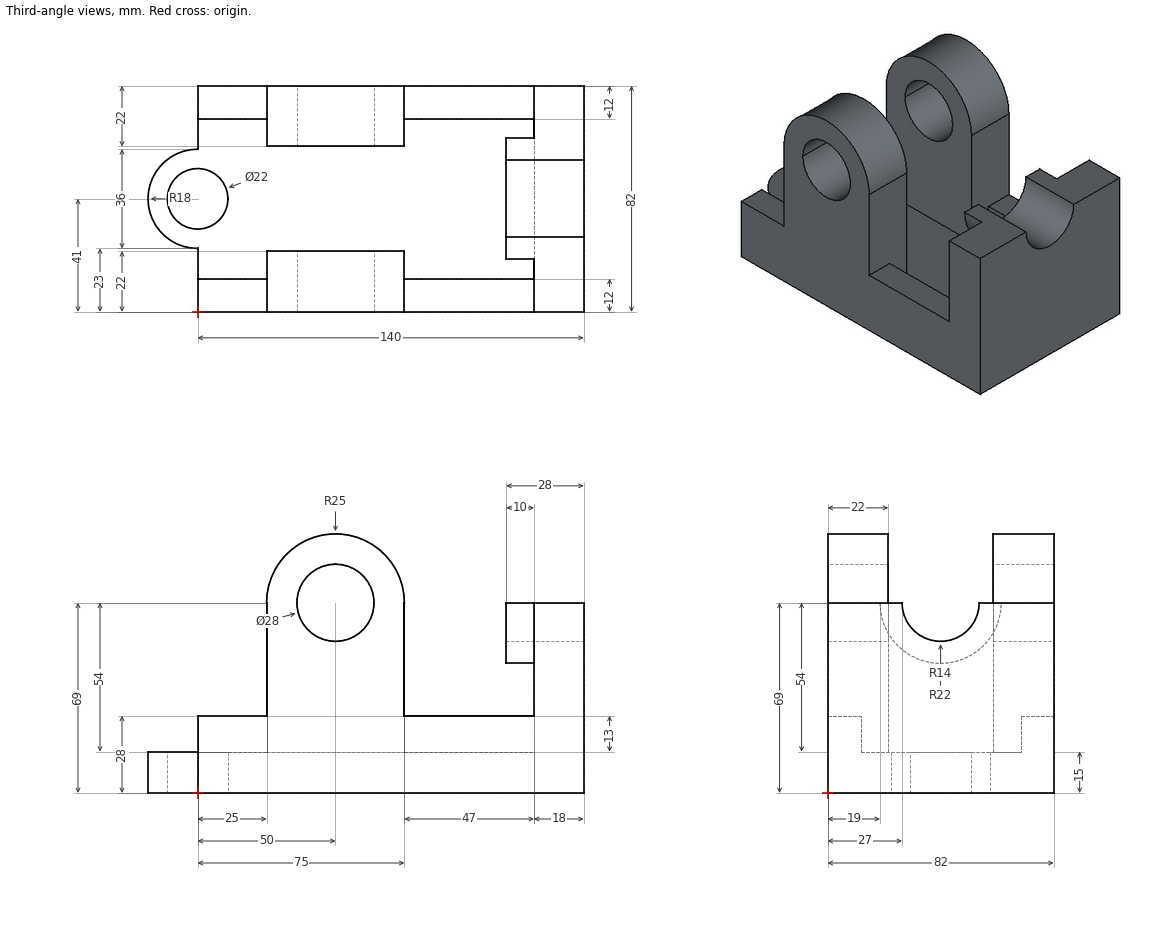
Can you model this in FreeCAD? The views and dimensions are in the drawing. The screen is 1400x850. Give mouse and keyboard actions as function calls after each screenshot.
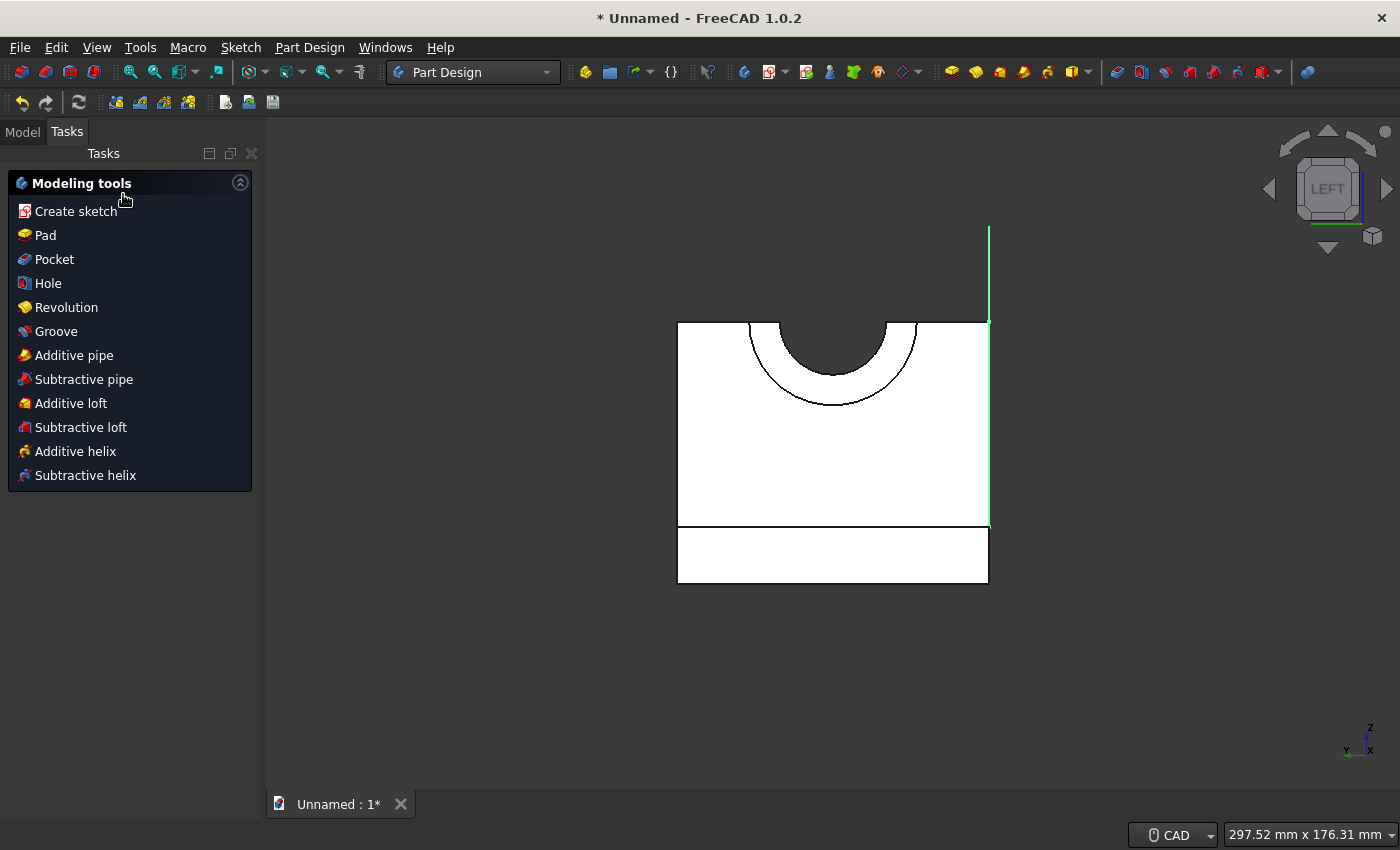
click(952, 72)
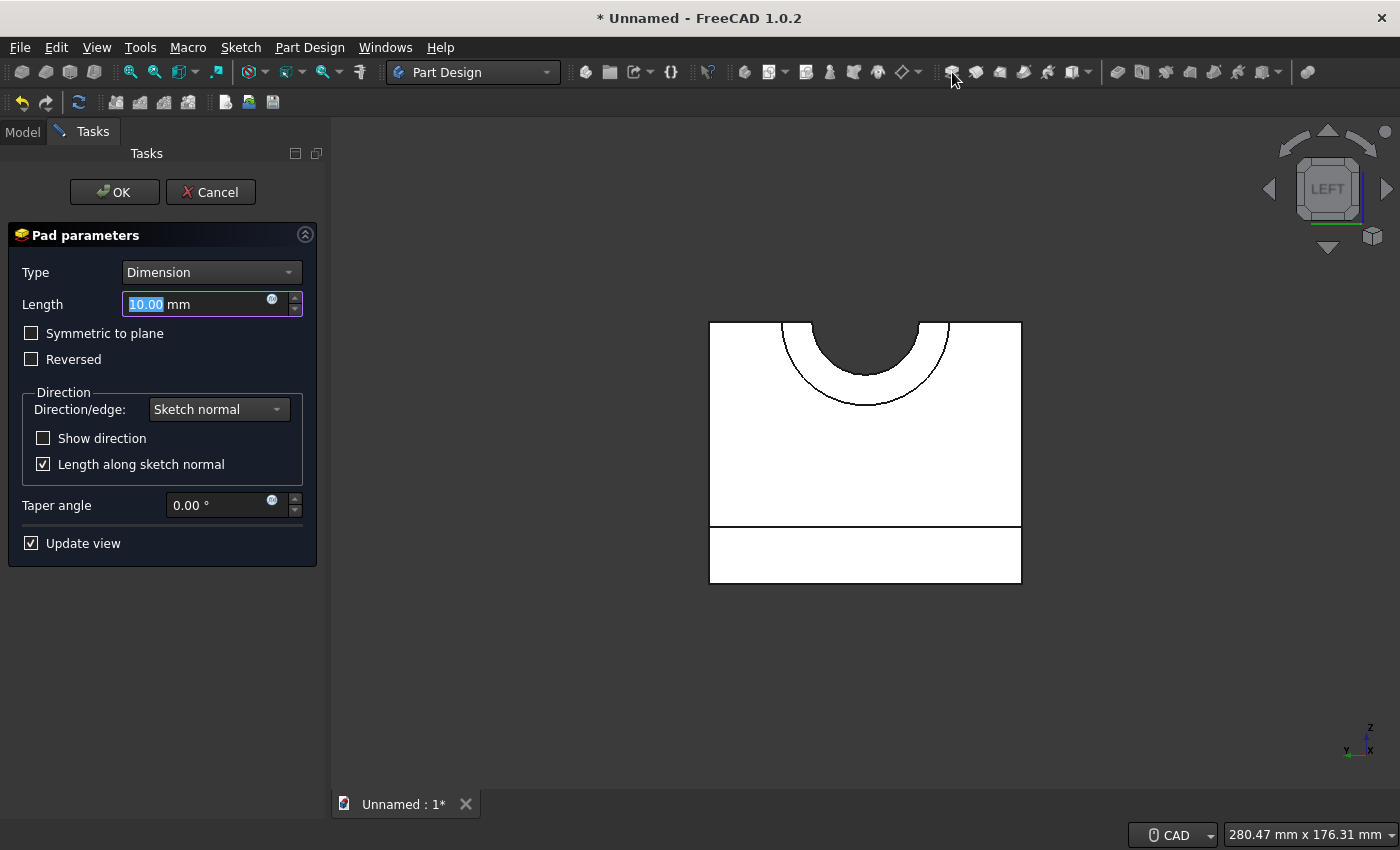
text(22)
key(Tab)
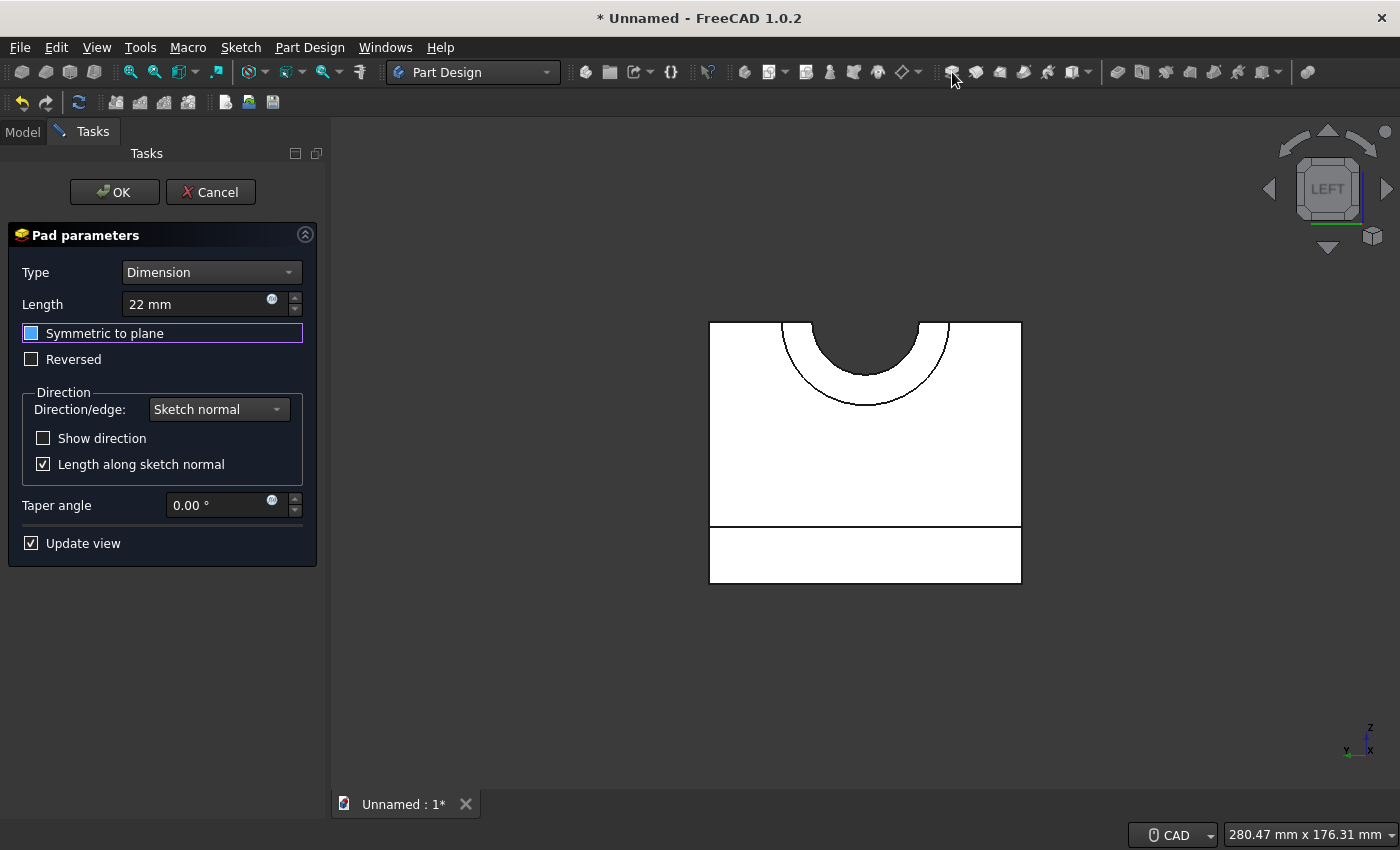
click(30, 359)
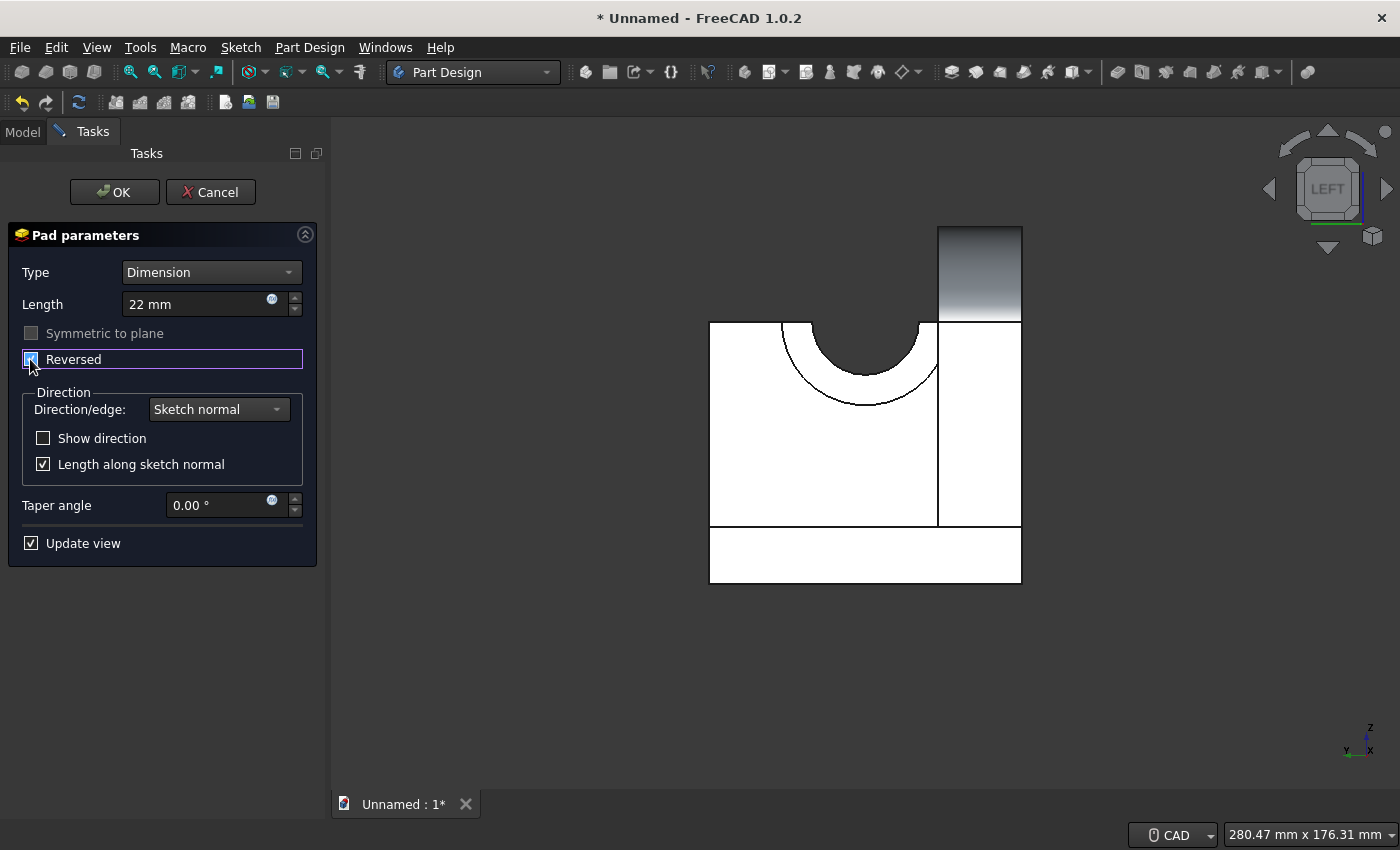
click(115, 192)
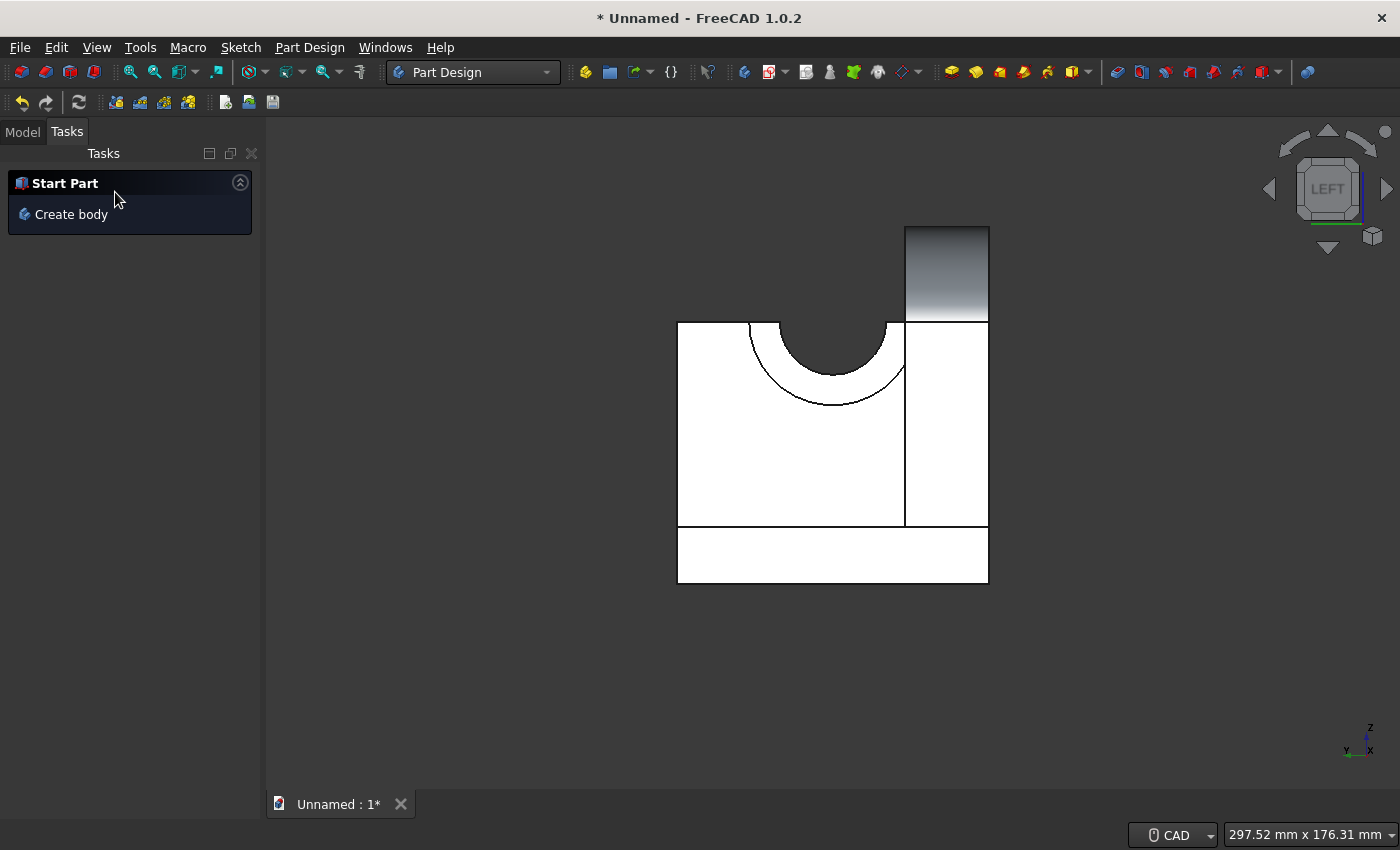
click(770, 72)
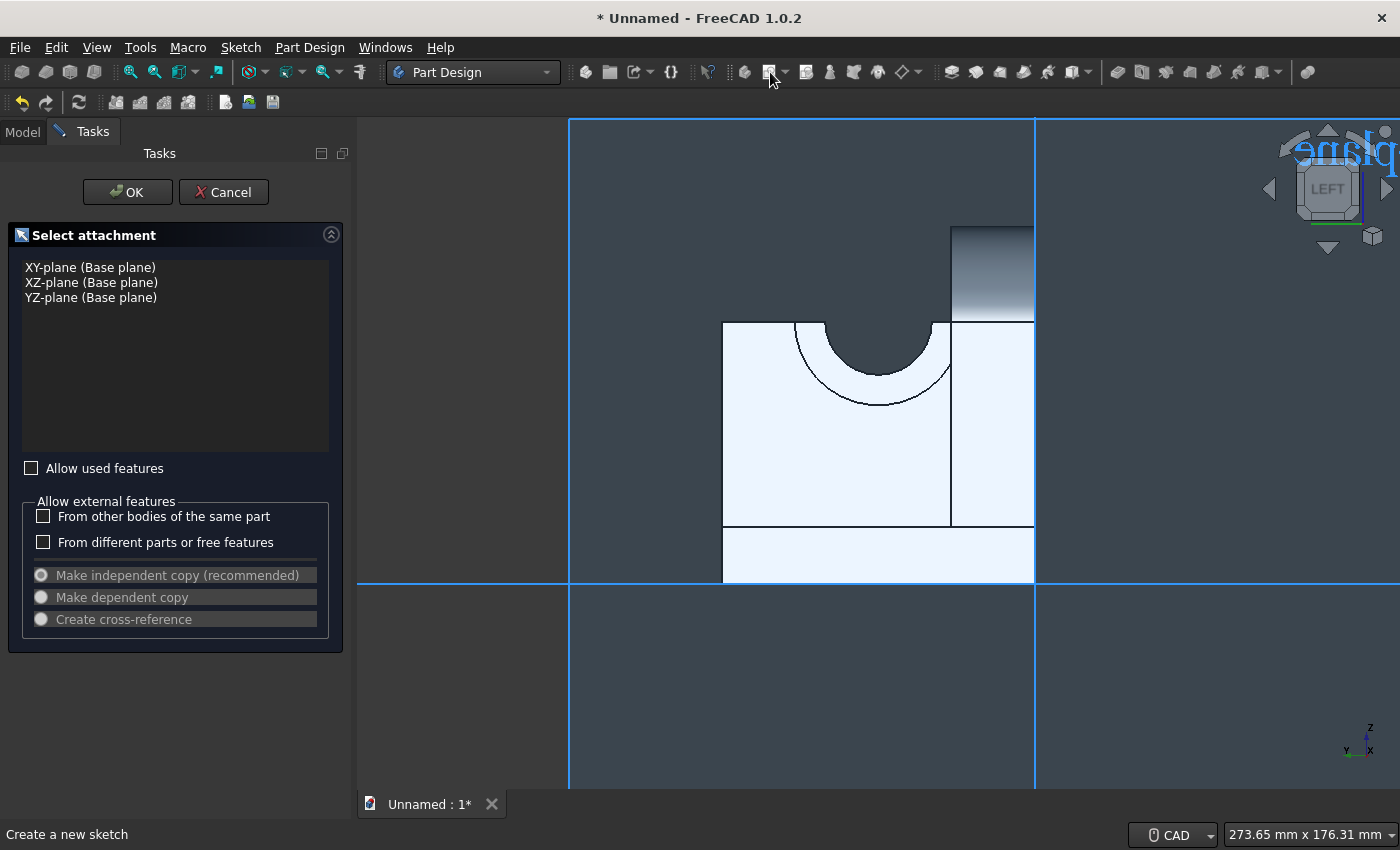
click(82, 282)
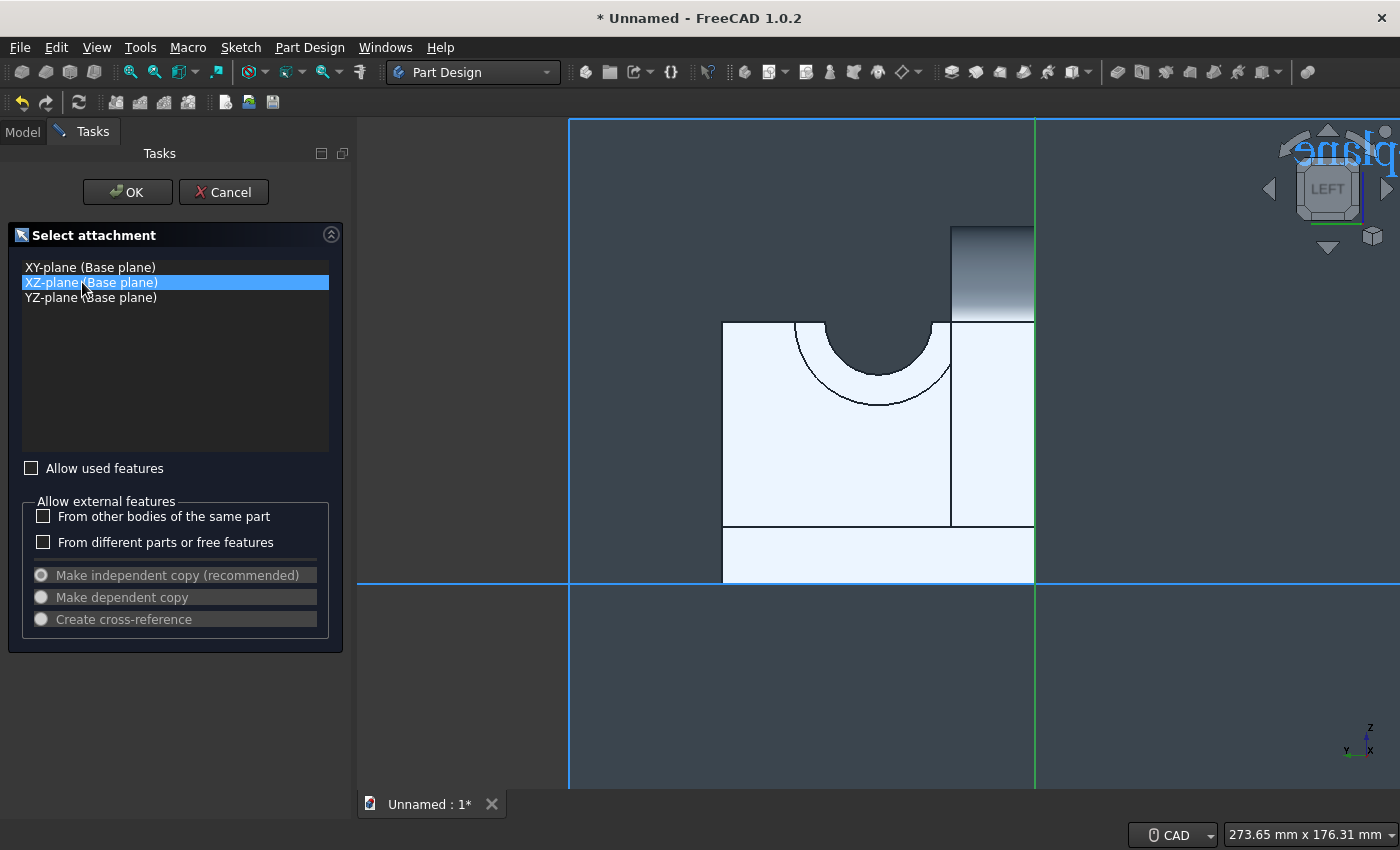
click(128, 192)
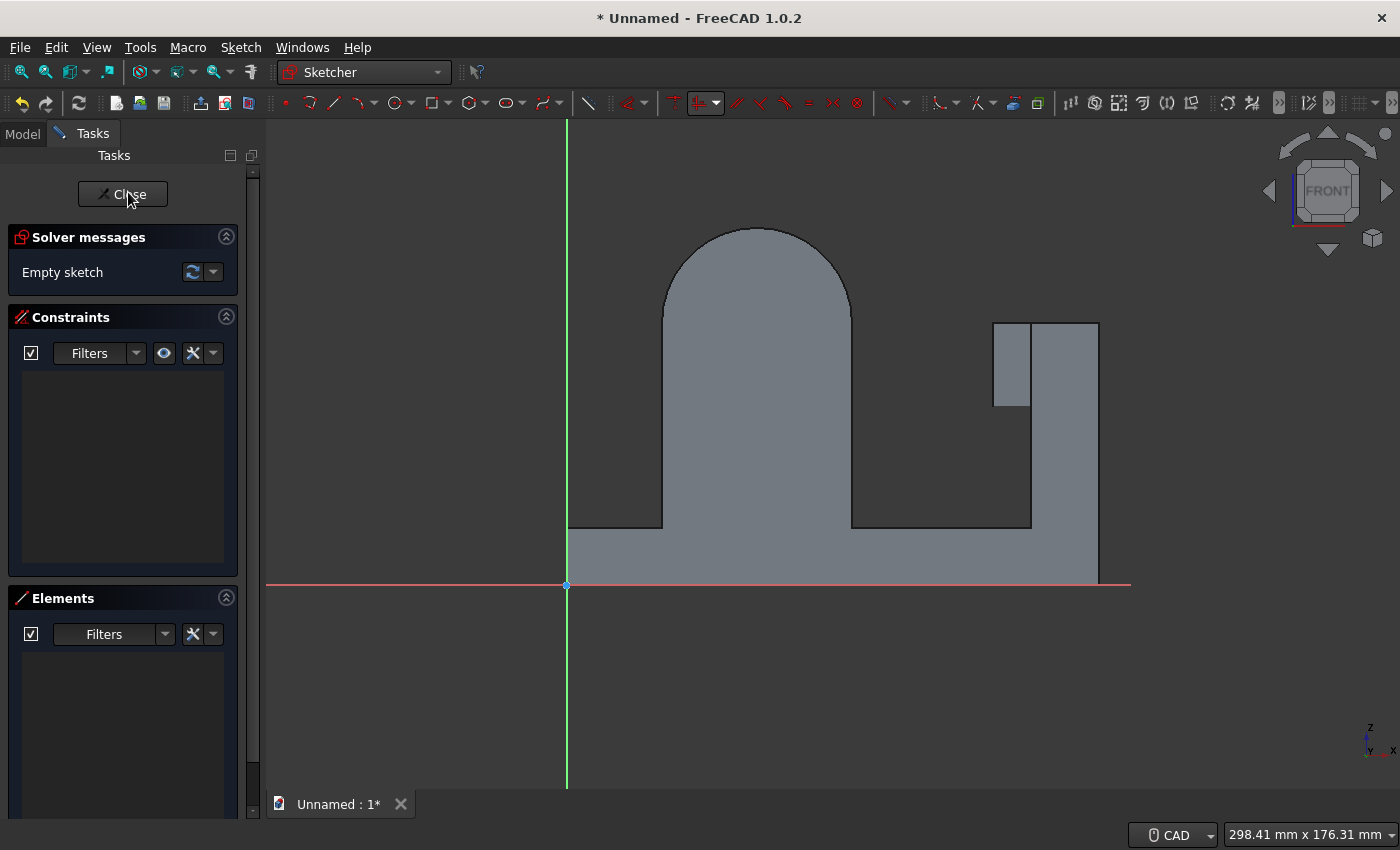
scroll(999, 520, up, 7)